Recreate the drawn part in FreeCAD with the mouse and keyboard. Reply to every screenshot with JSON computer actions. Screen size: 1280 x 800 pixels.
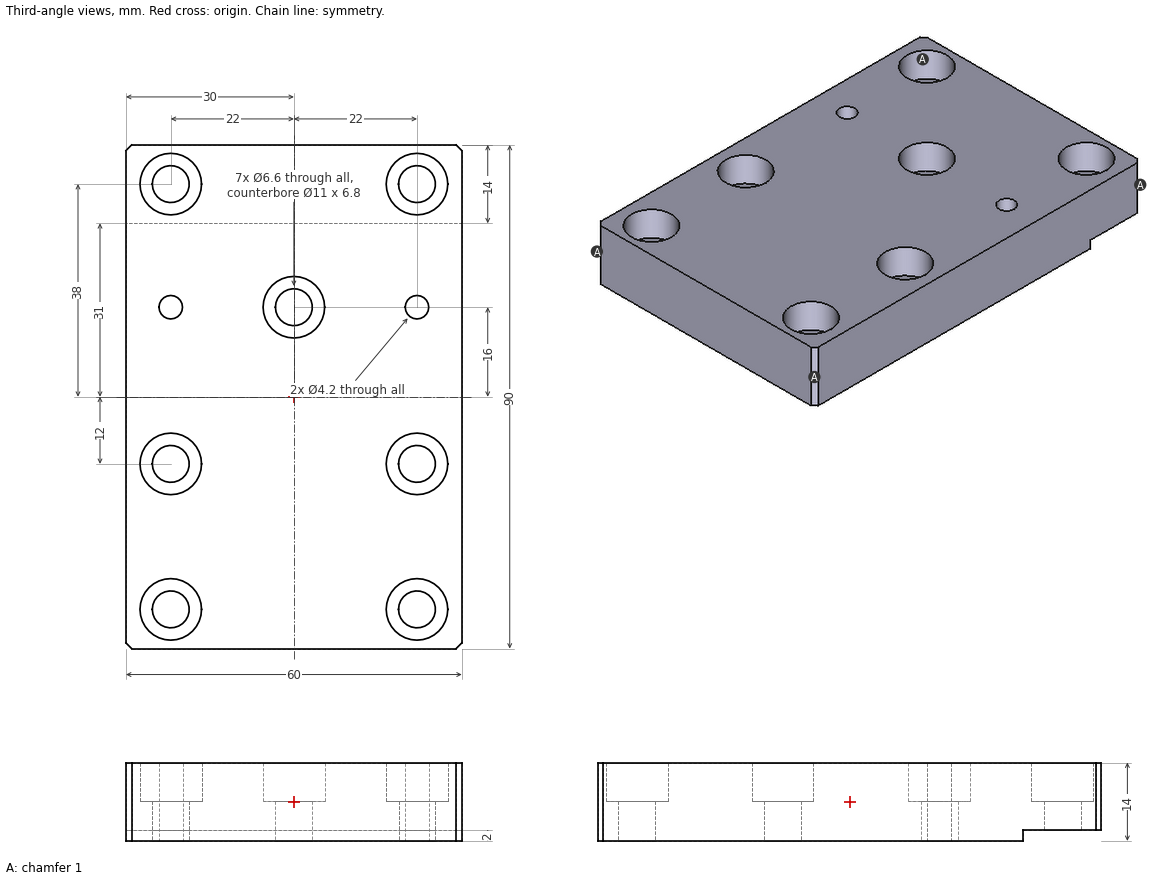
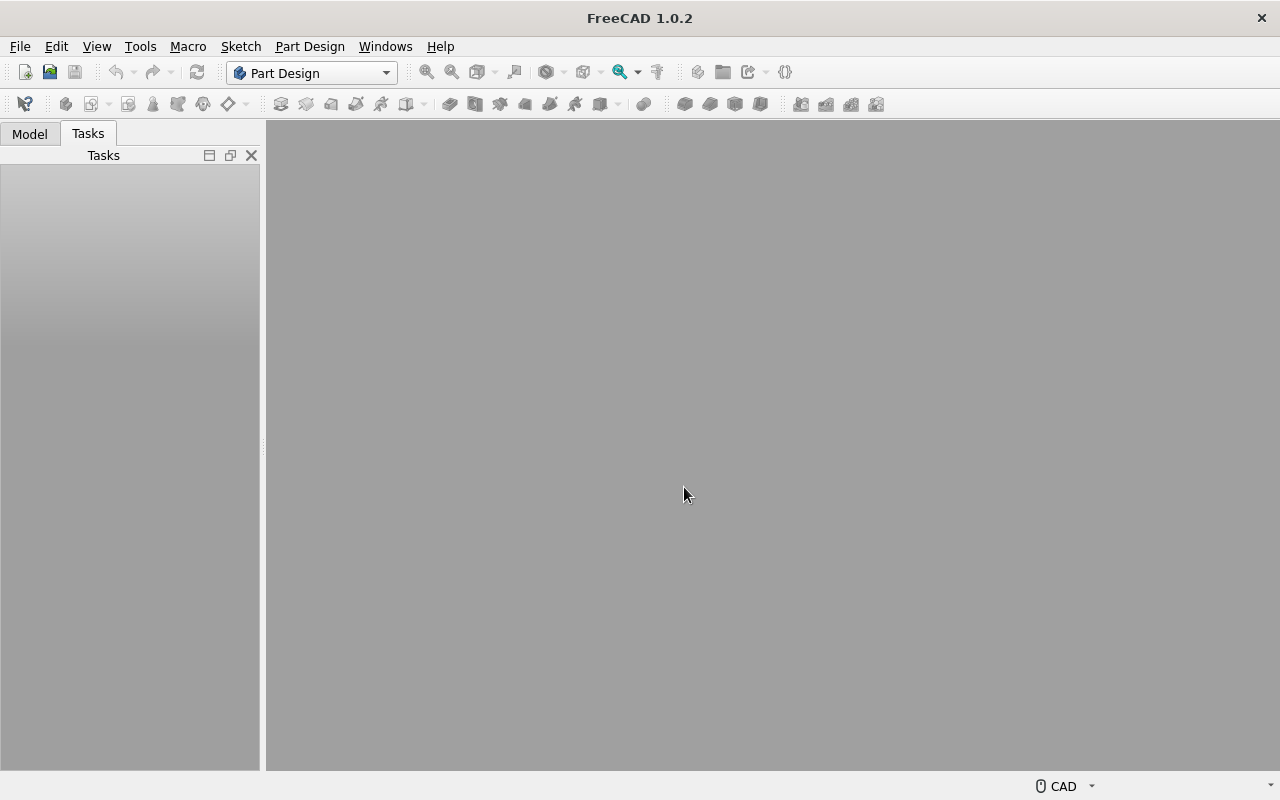
{"action": "left_click", "coordinate": [25, 72]}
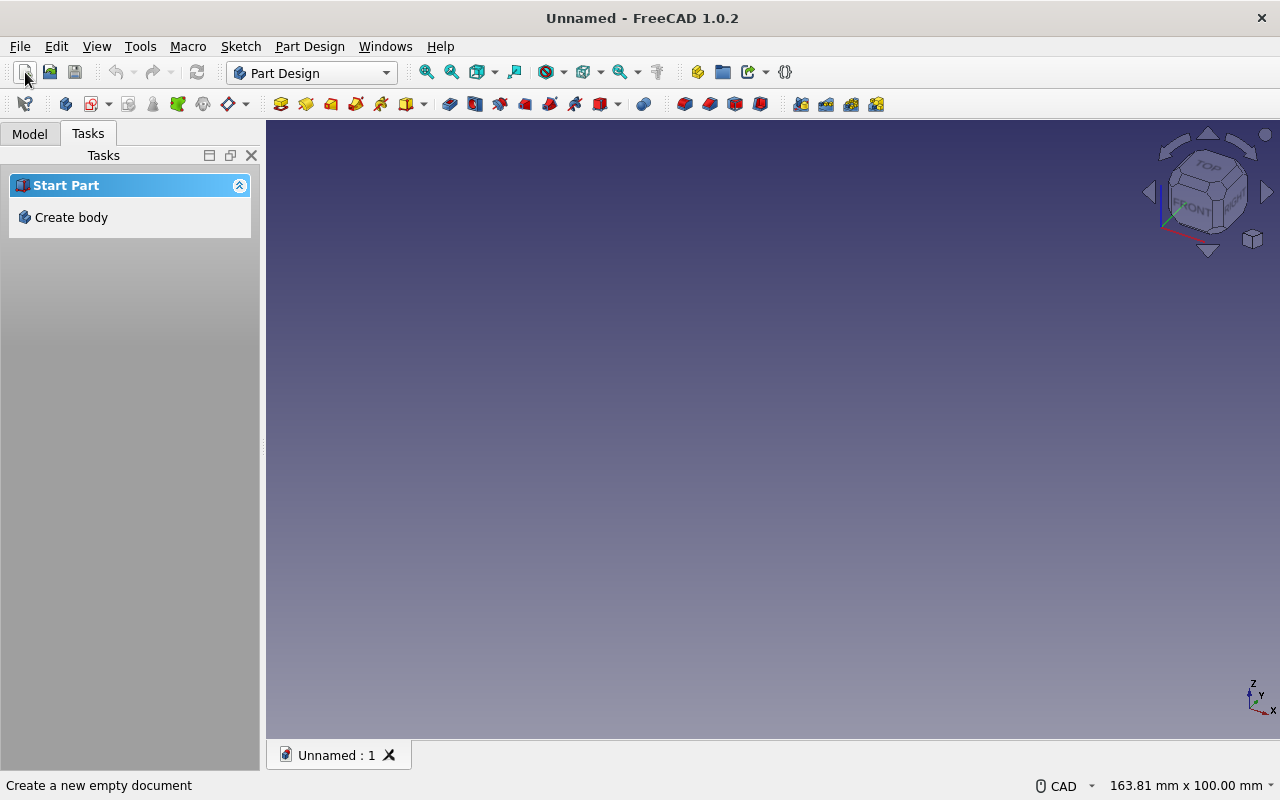
{"action": "left_click", "coordinate": [90, 104]}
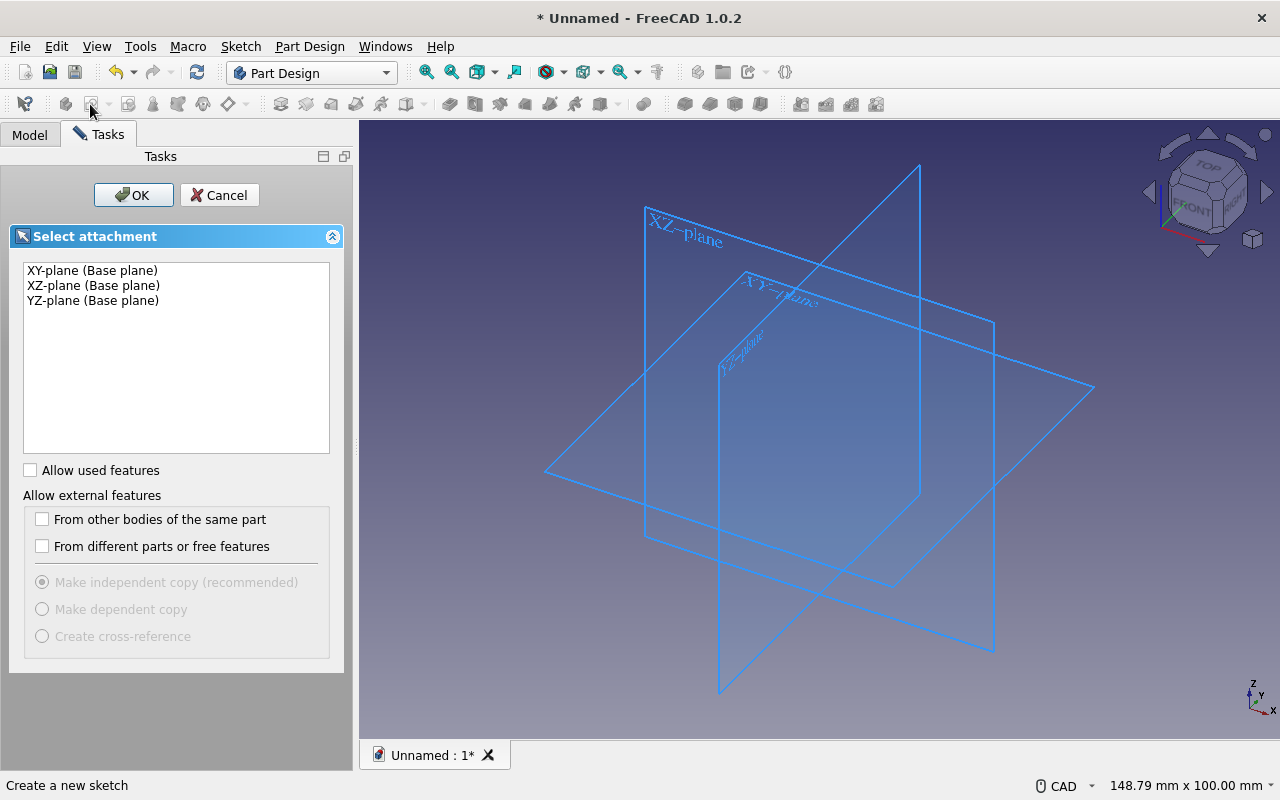
{"action": "left_click", "coordinate": [84, 270]}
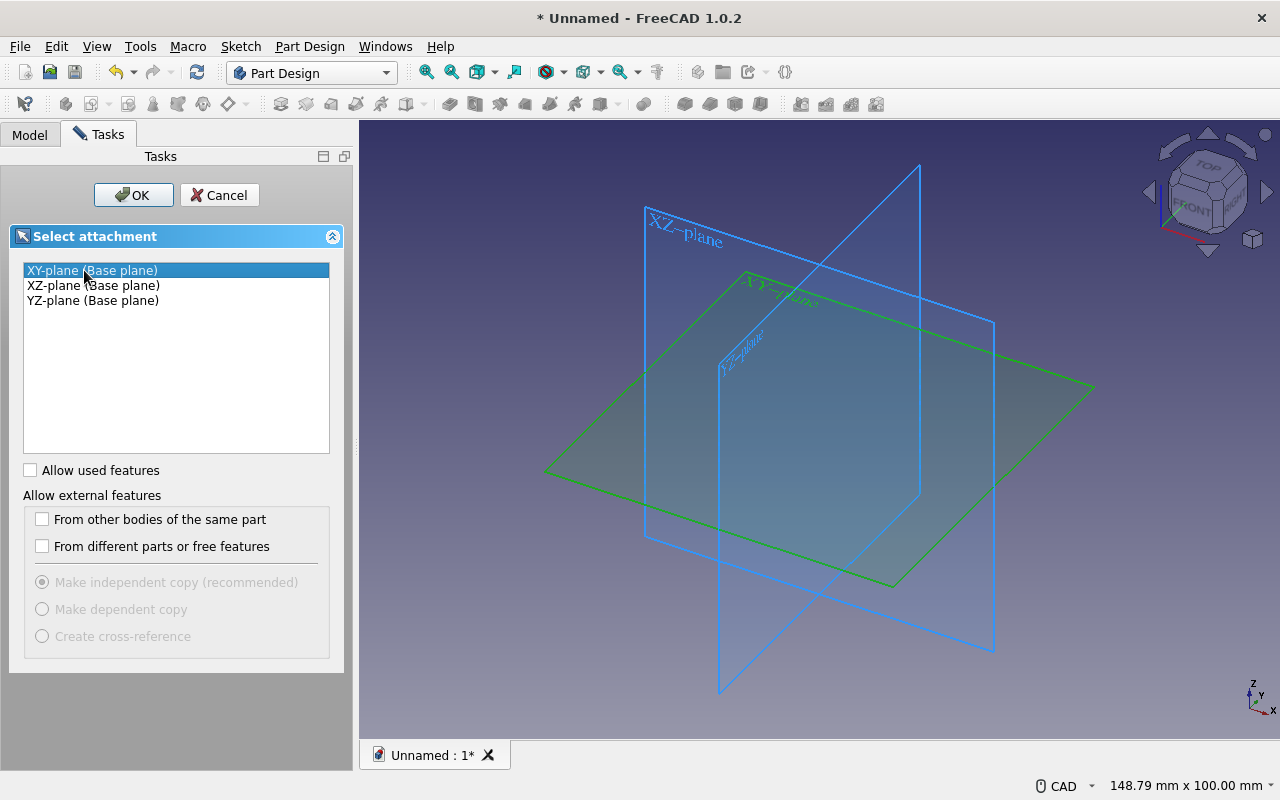
{"action": "left_click", "coordinate": [134, 195]}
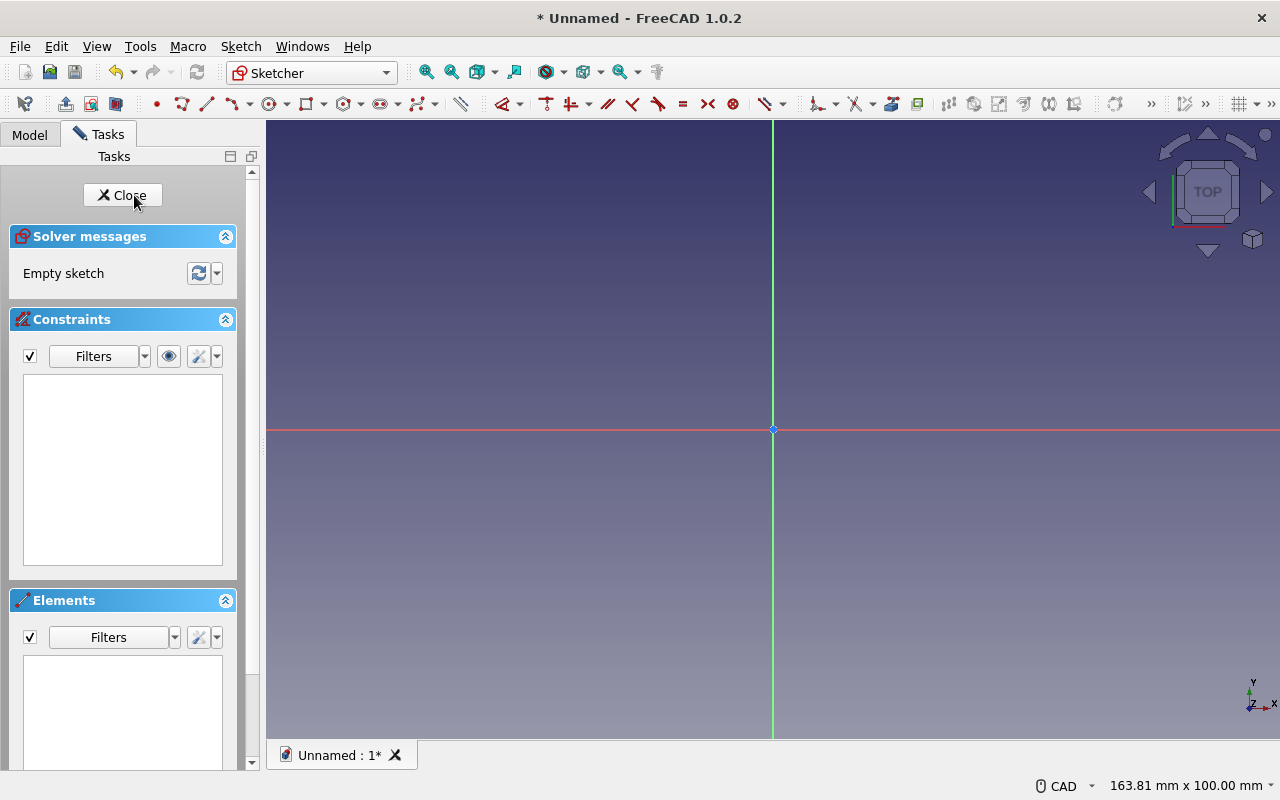
{"action": "scroll", "coordinate": [565, 429], "scroll_direction": "down", "scroll_amount": 2}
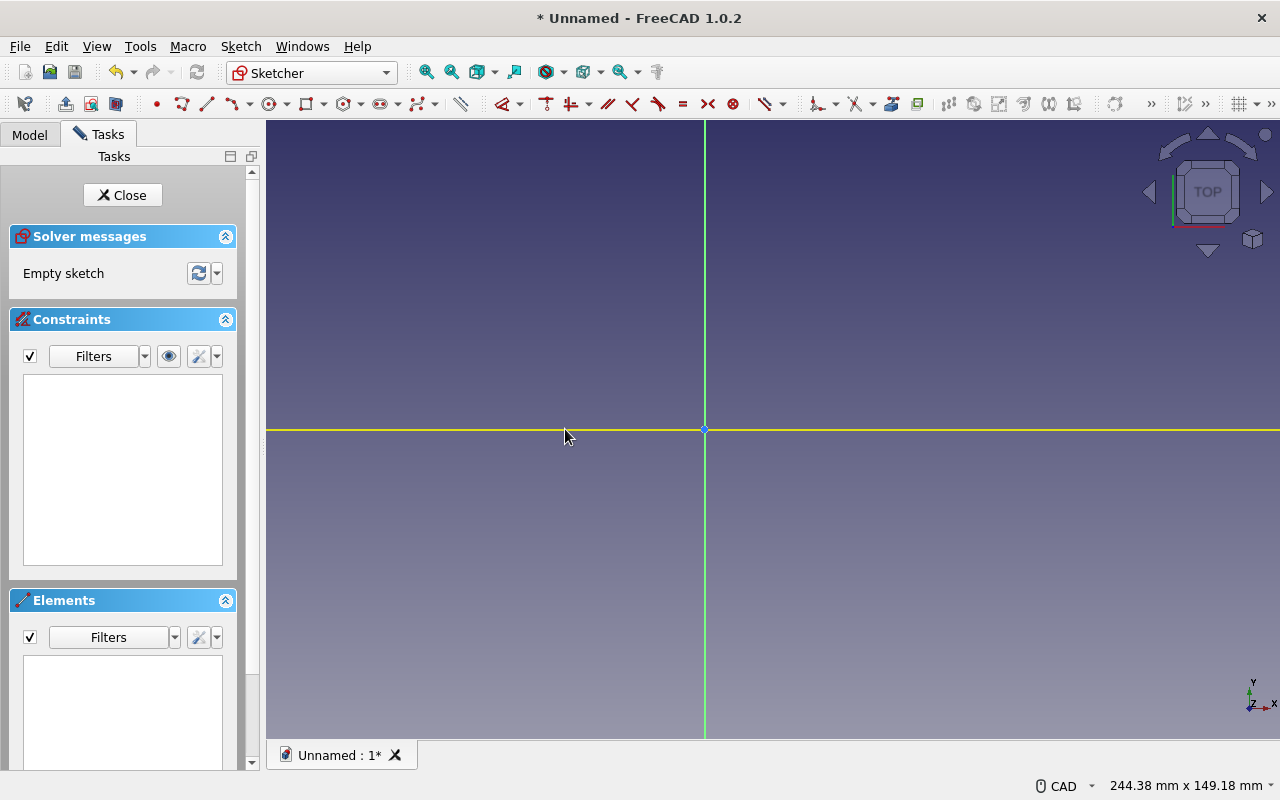
{"action": "left_click", "coordinate": [324, 104]}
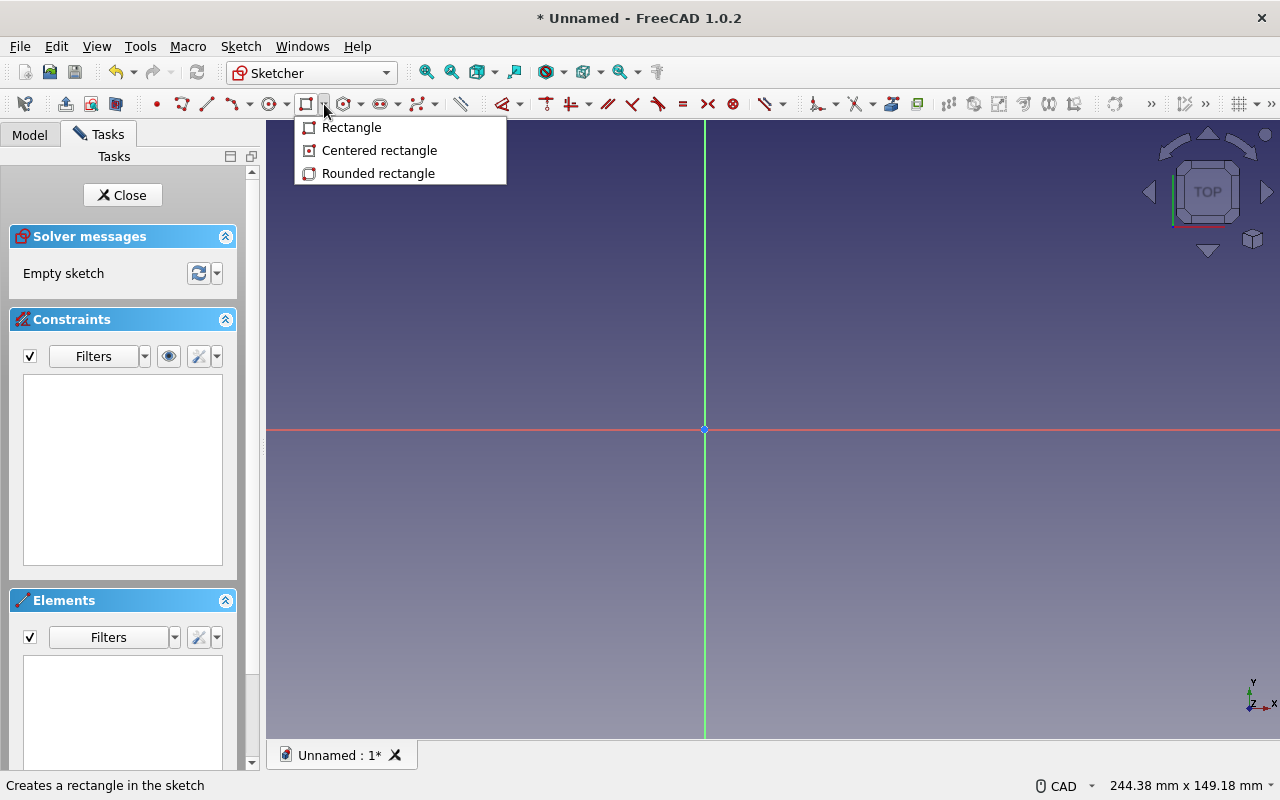
{"action": "left_click", "coordinate": [400, 150]}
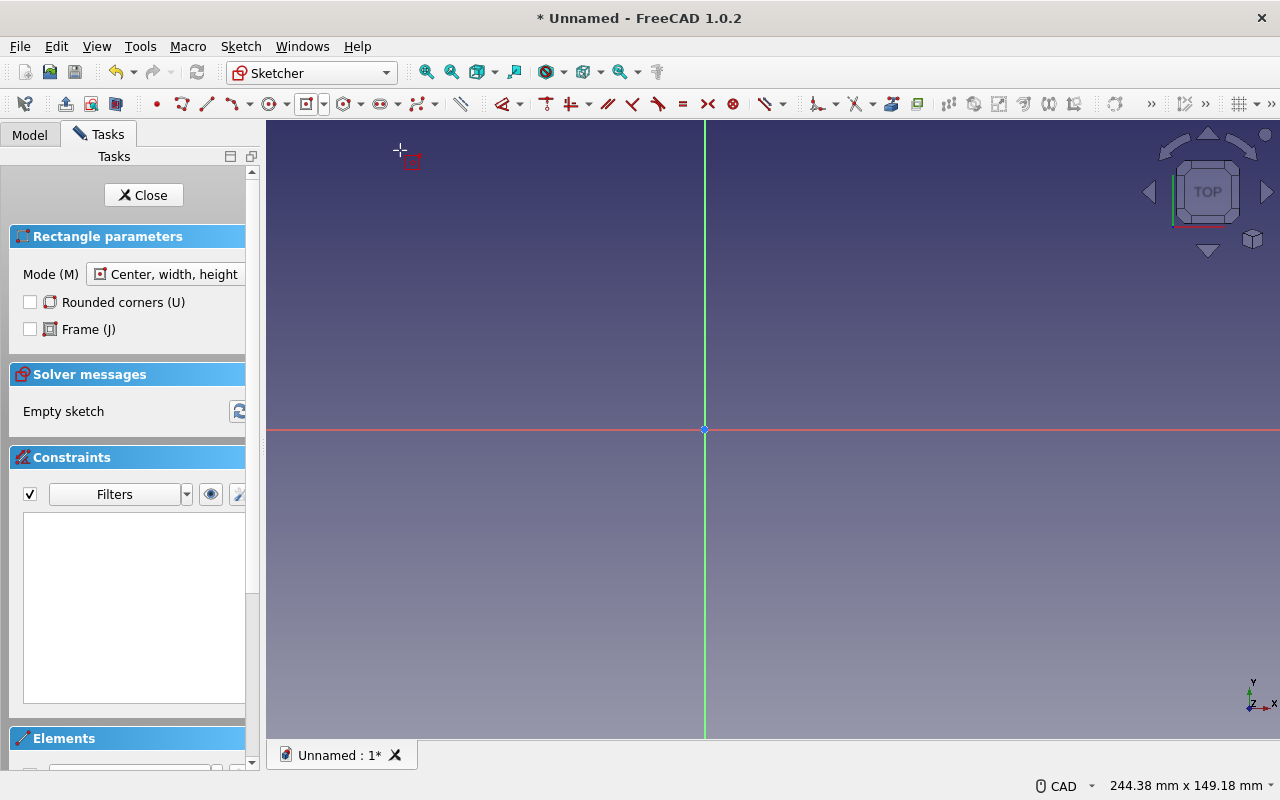
{"action": "left_click", "coordinate": [705, 430]}
{"action": "mouse_move", "coordinate": [829, 243]}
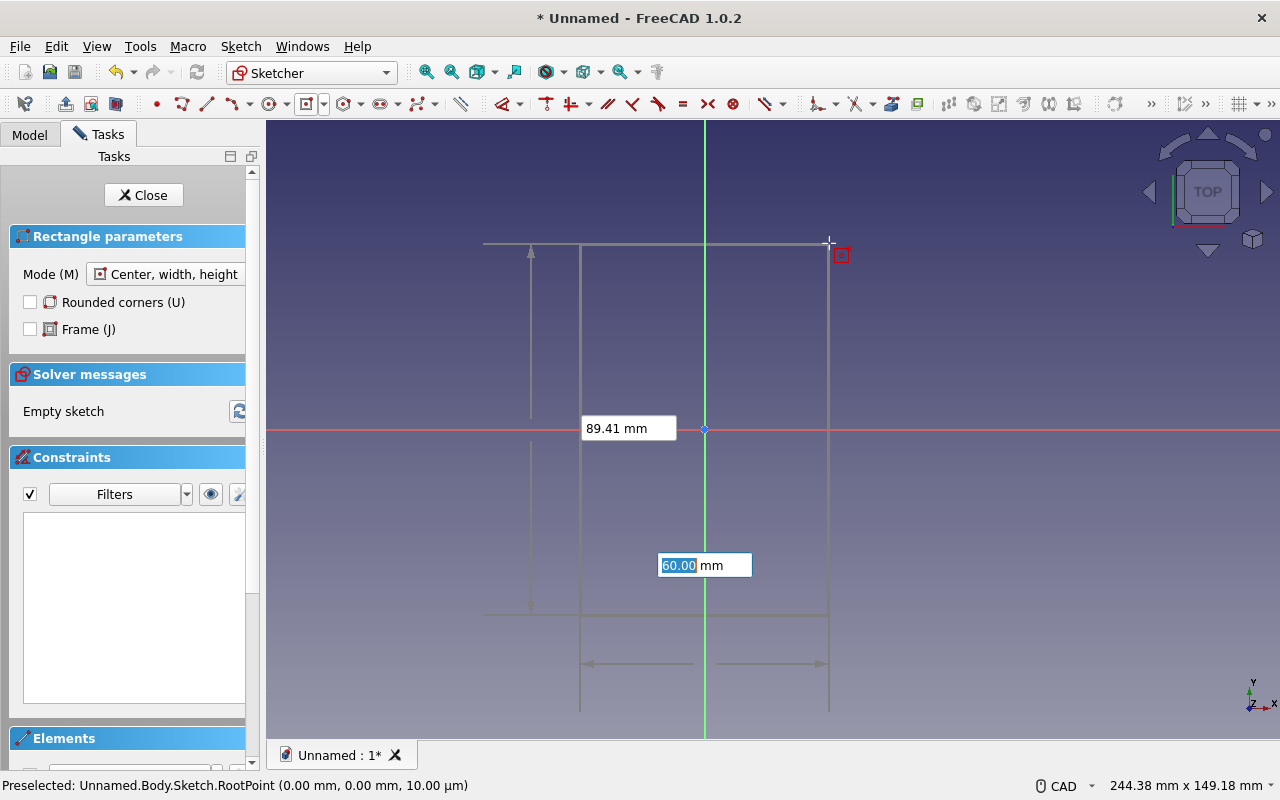
{"action": "type", "text": "60"}
{"action": "key", "text": "Tab"}
{"action": "type", "text": "90"}
{"action": "key", "text": "Return"}
{"action": "key", "text": "Escape"}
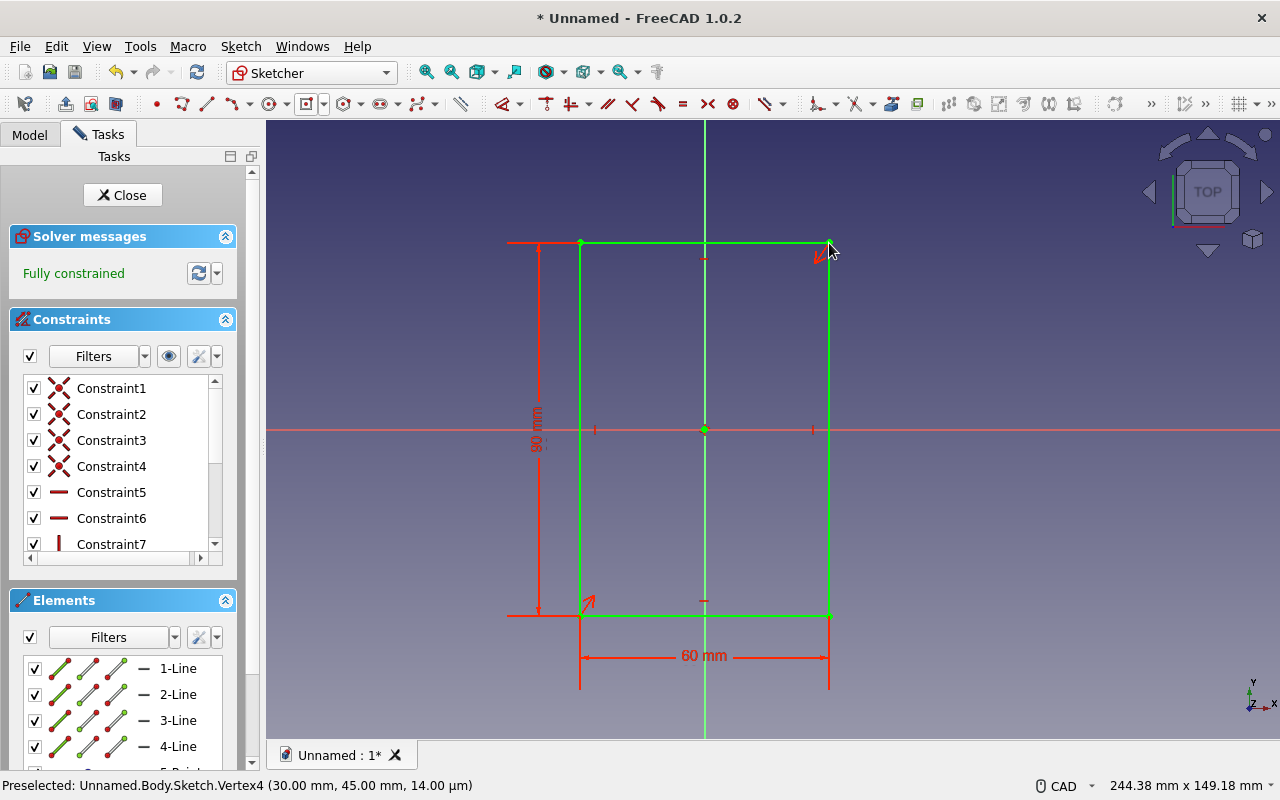
{"action": "left_click", "coordinate": [123, 195]}